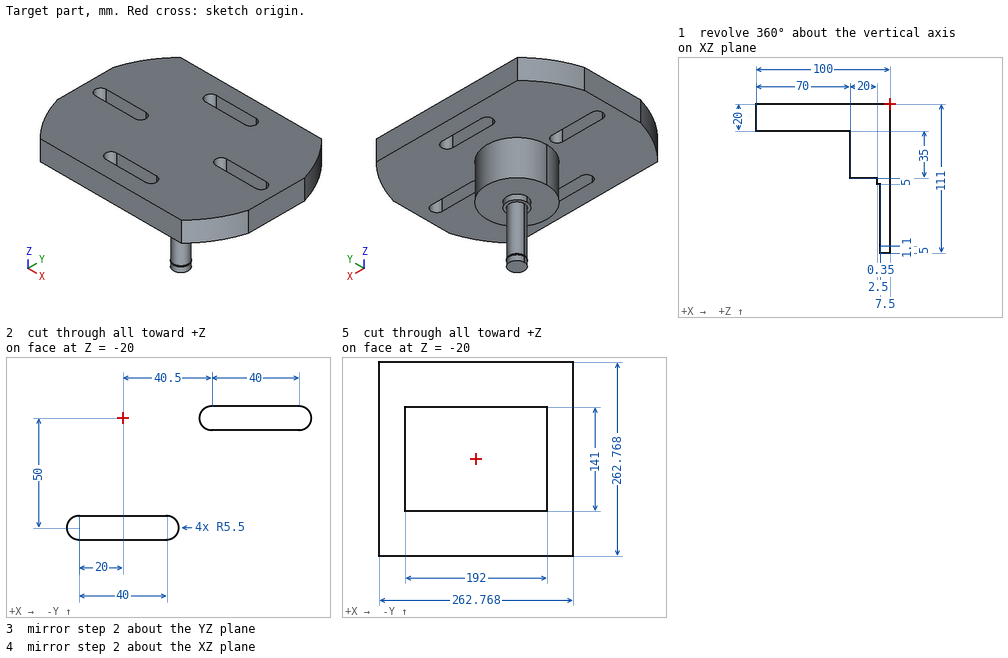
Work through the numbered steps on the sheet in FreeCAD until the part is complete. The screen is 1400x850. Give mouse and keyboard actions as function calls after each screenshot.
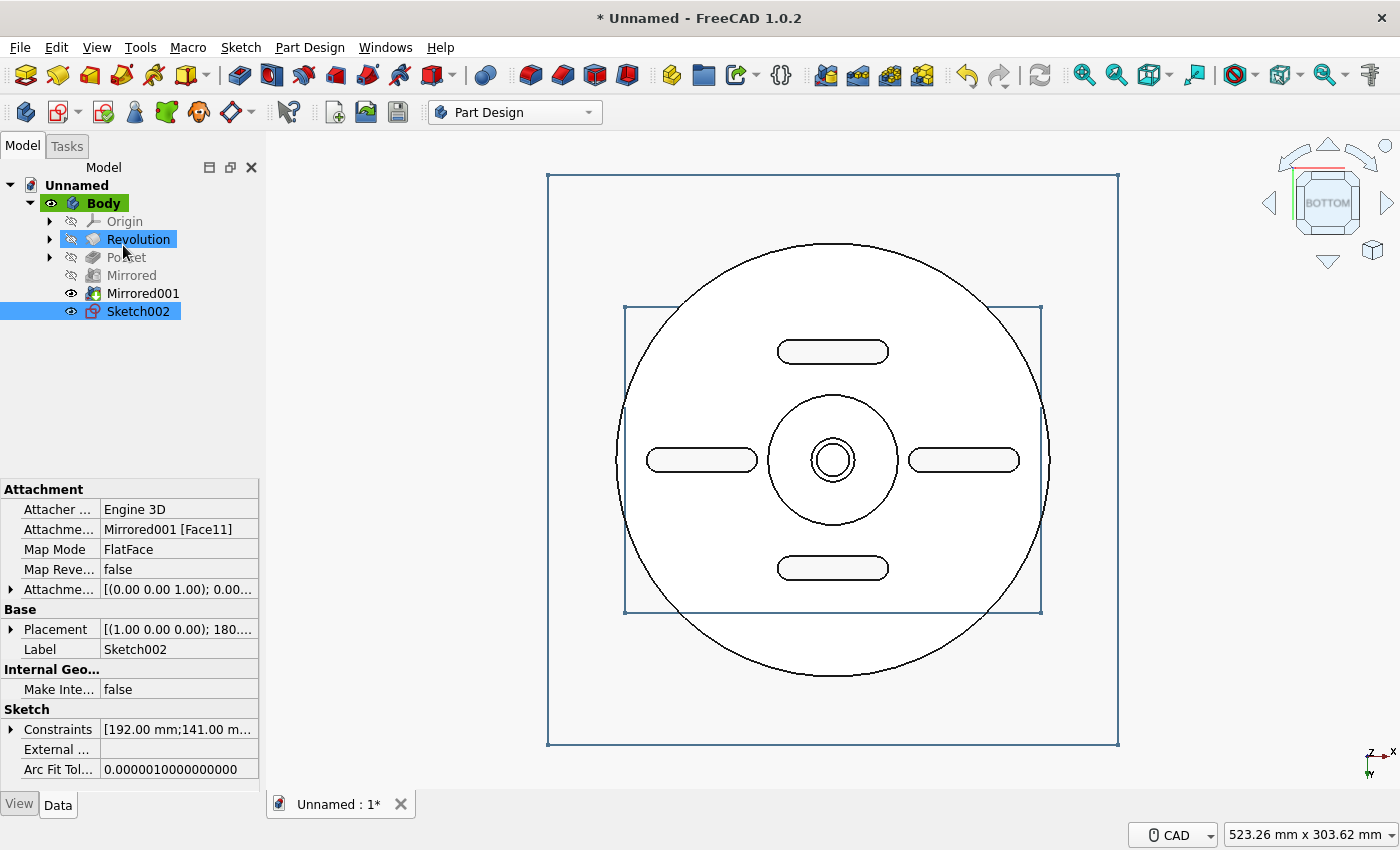
click(240, 76)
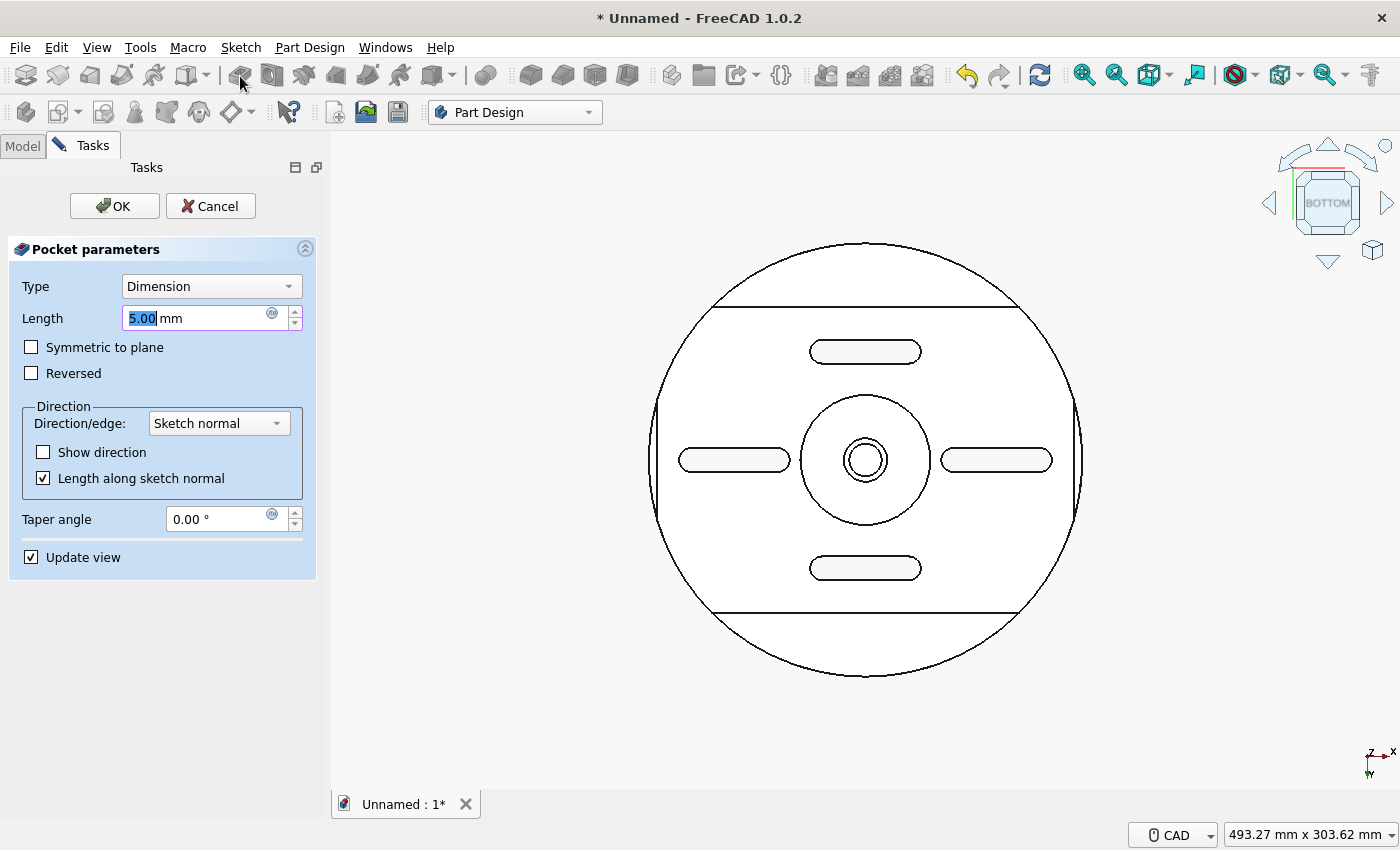
click(212, 286)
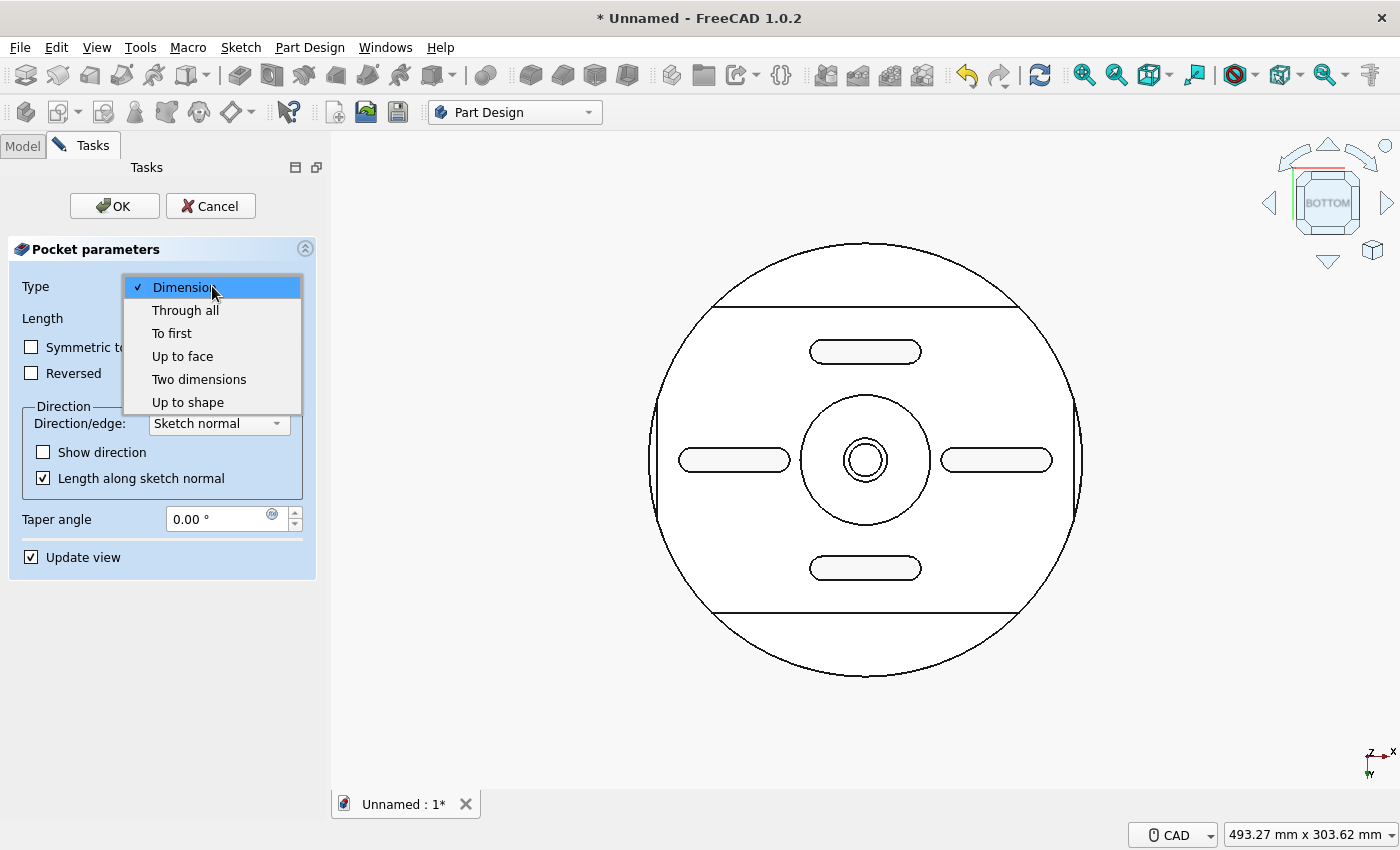
click(212, 310)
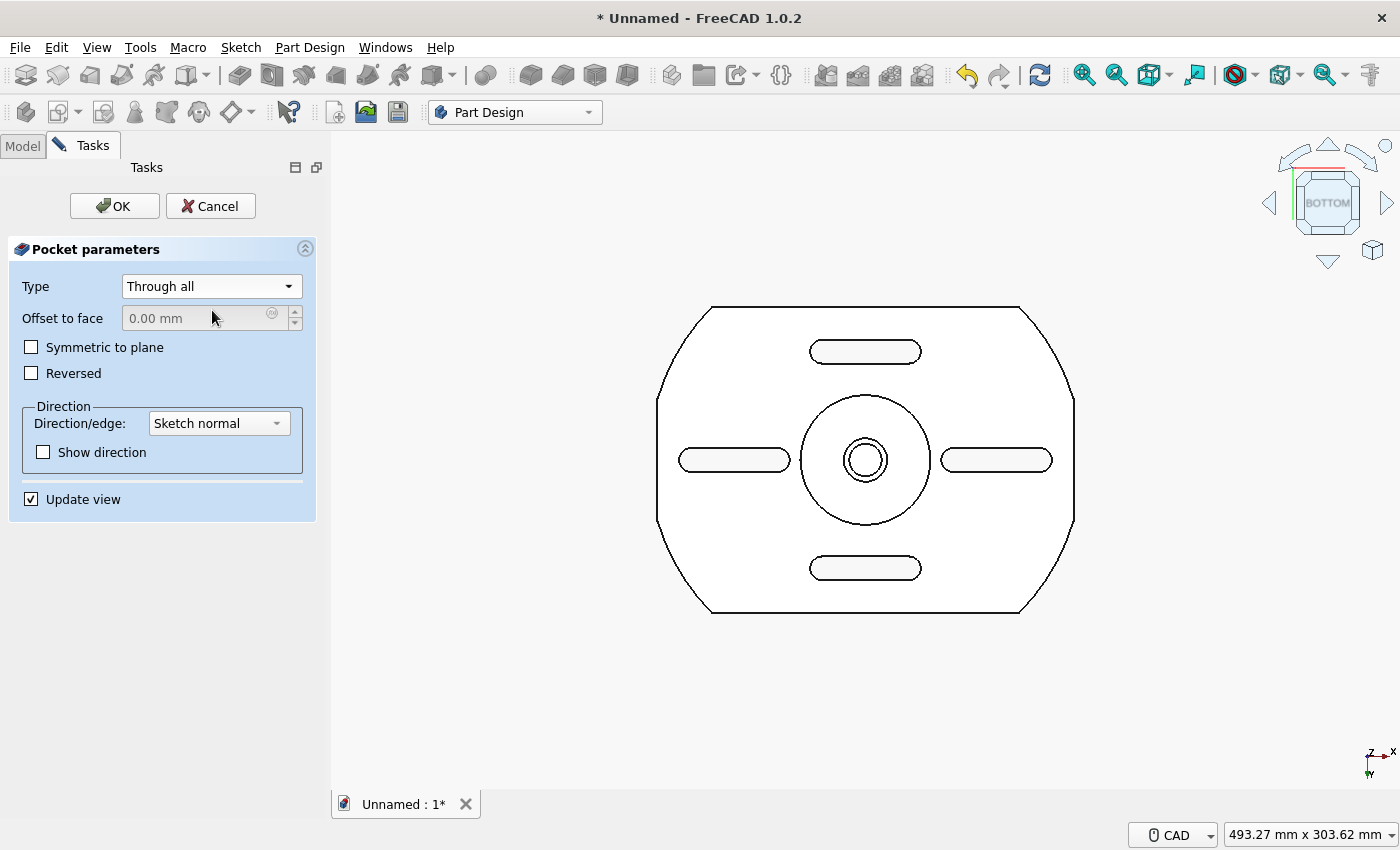
click(115, 206)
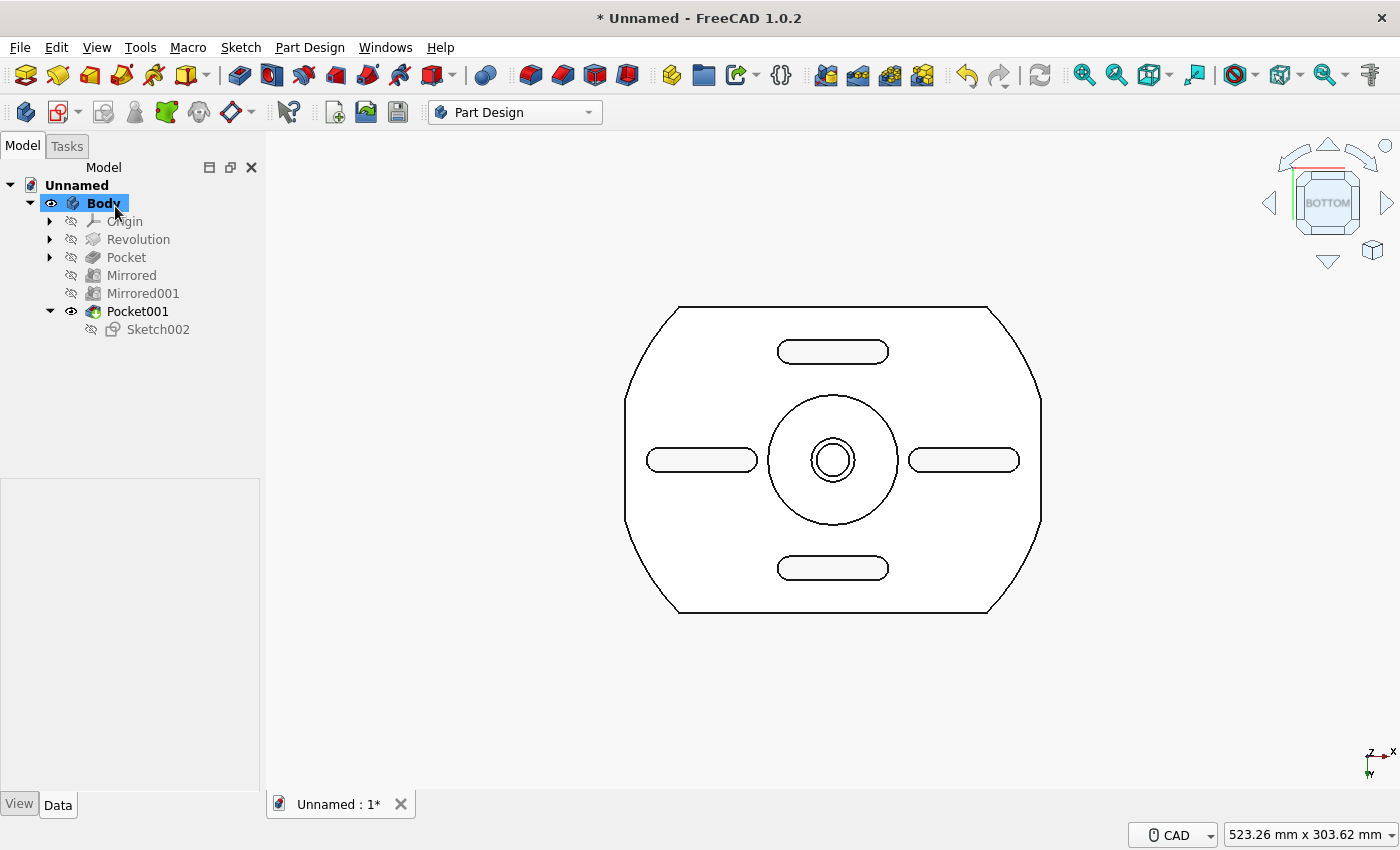
key(0)